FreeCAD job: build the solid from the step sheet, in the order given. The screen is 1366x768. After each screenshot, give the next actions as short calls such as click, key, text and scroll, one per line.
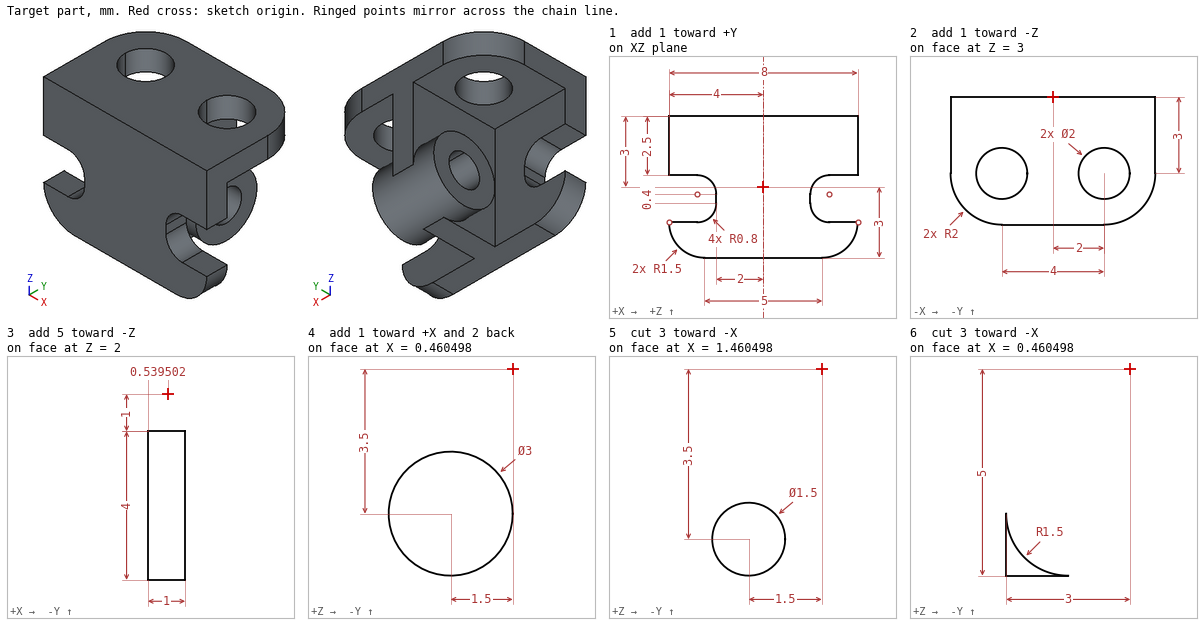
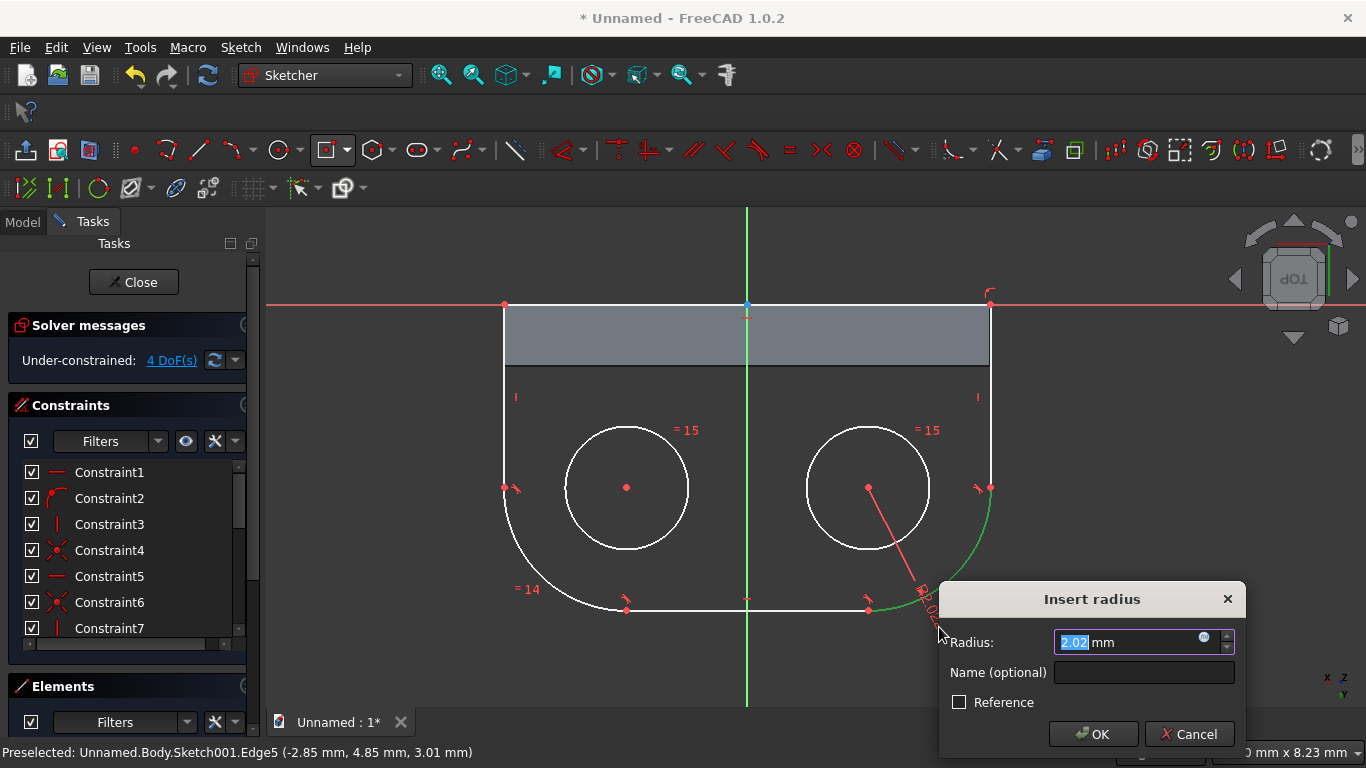
text(2)
key(Return)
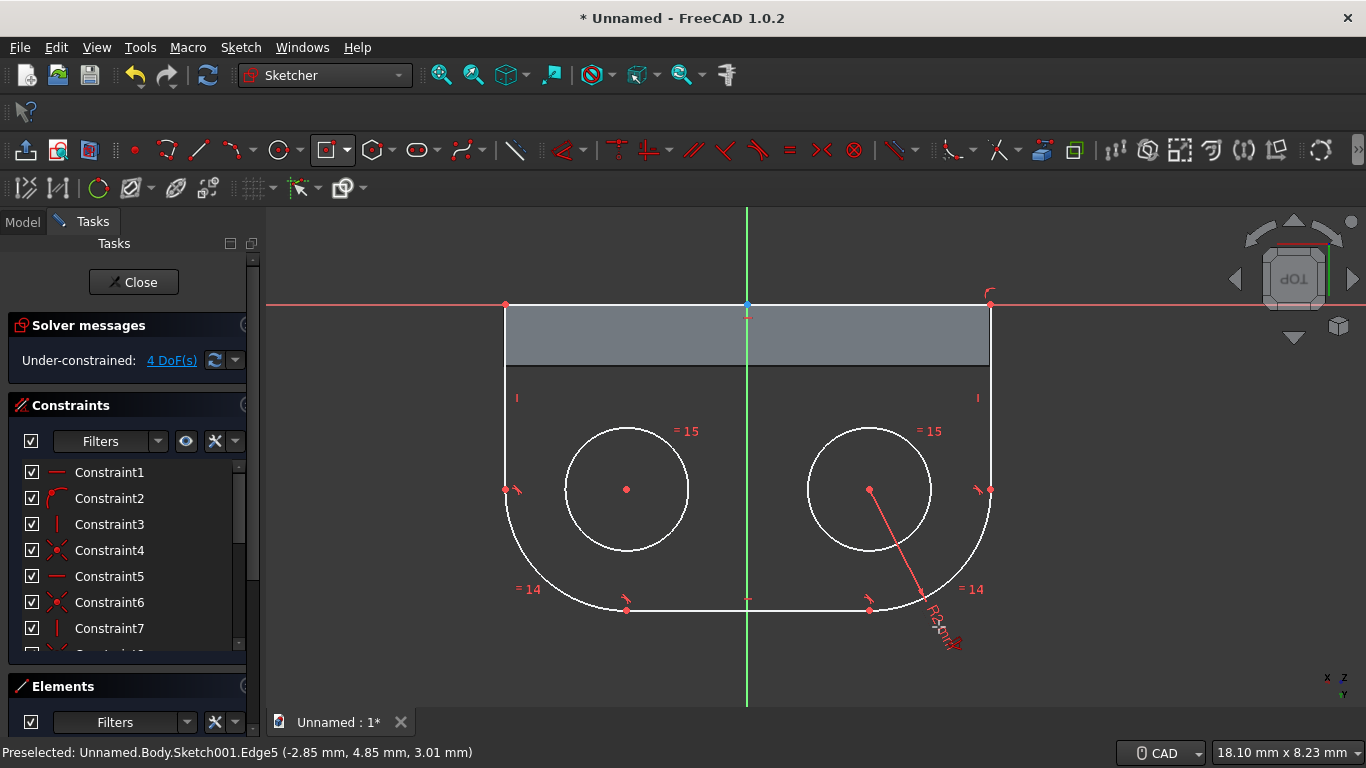
click(913, 446)
click(936, 423)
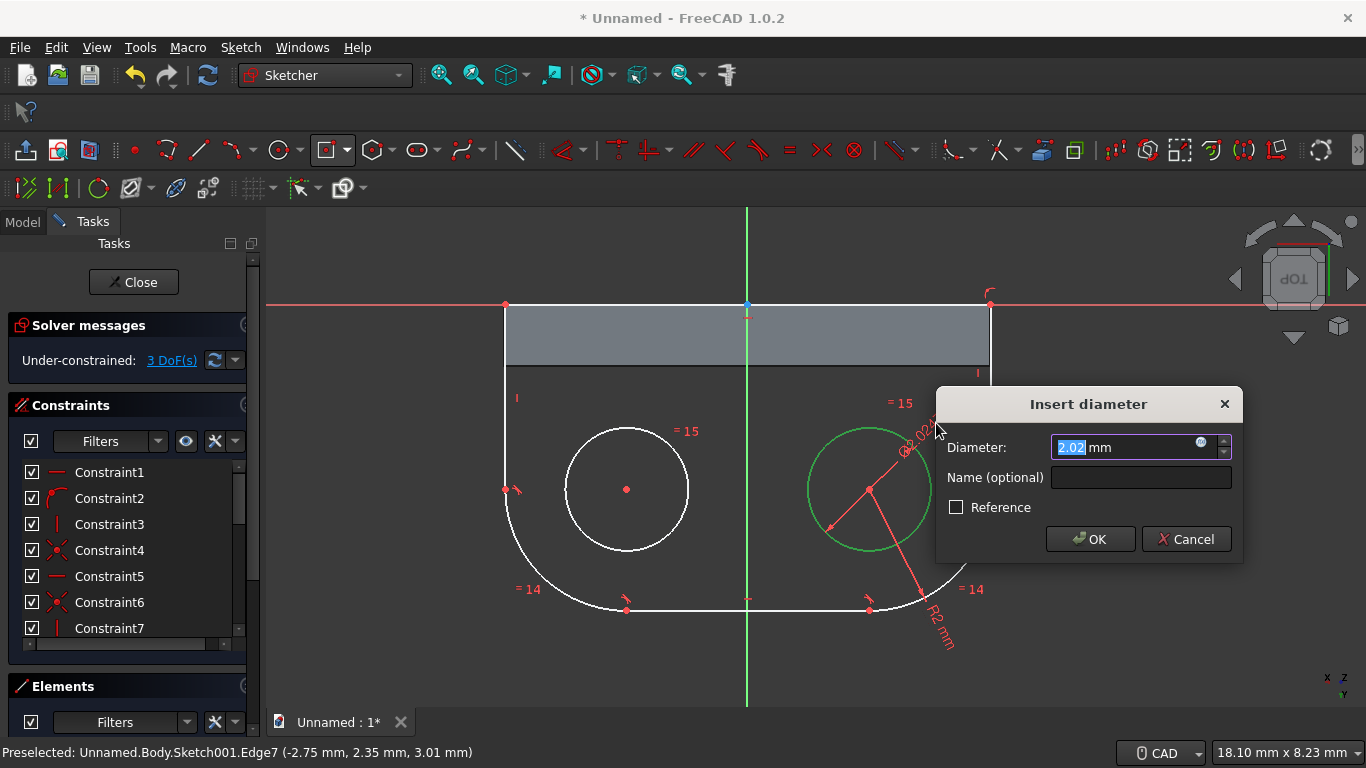
text(2)
key(Return)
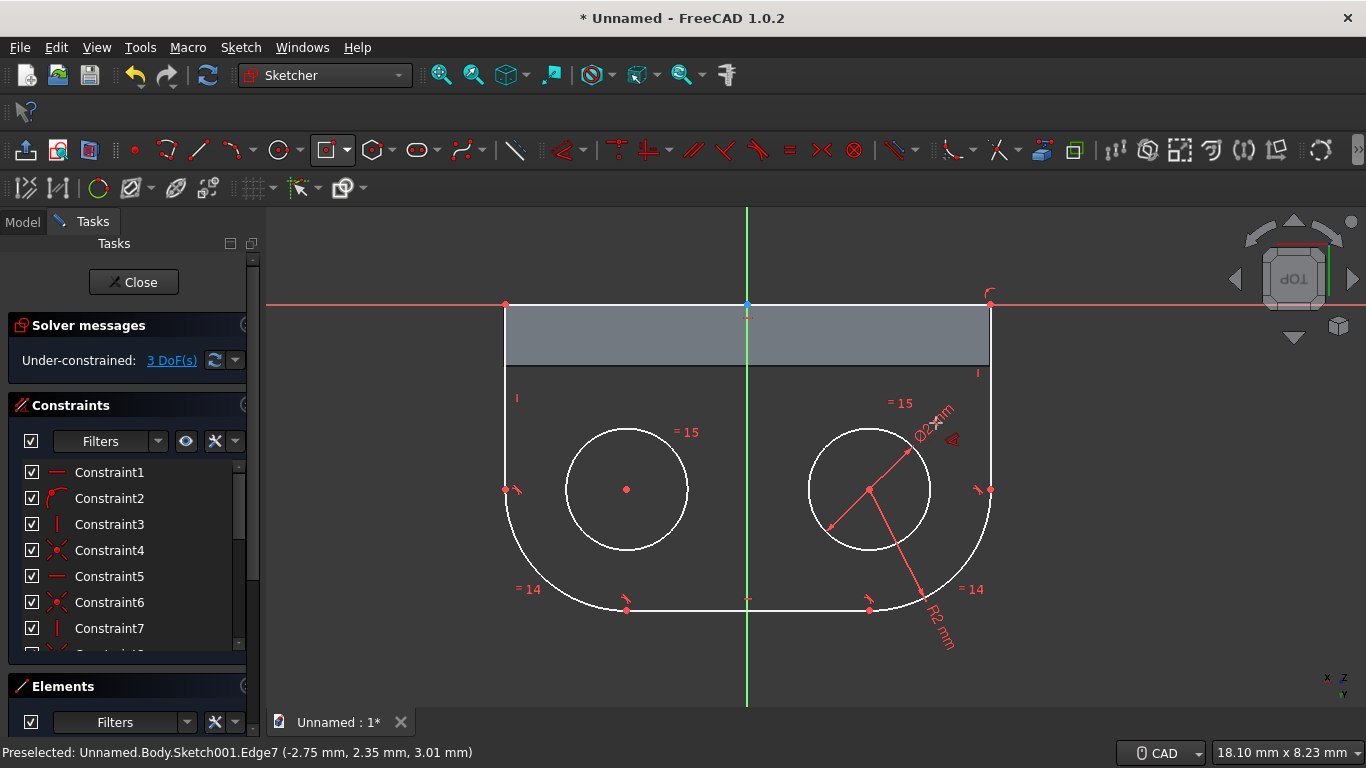
click(700, 611)
click(692, 645)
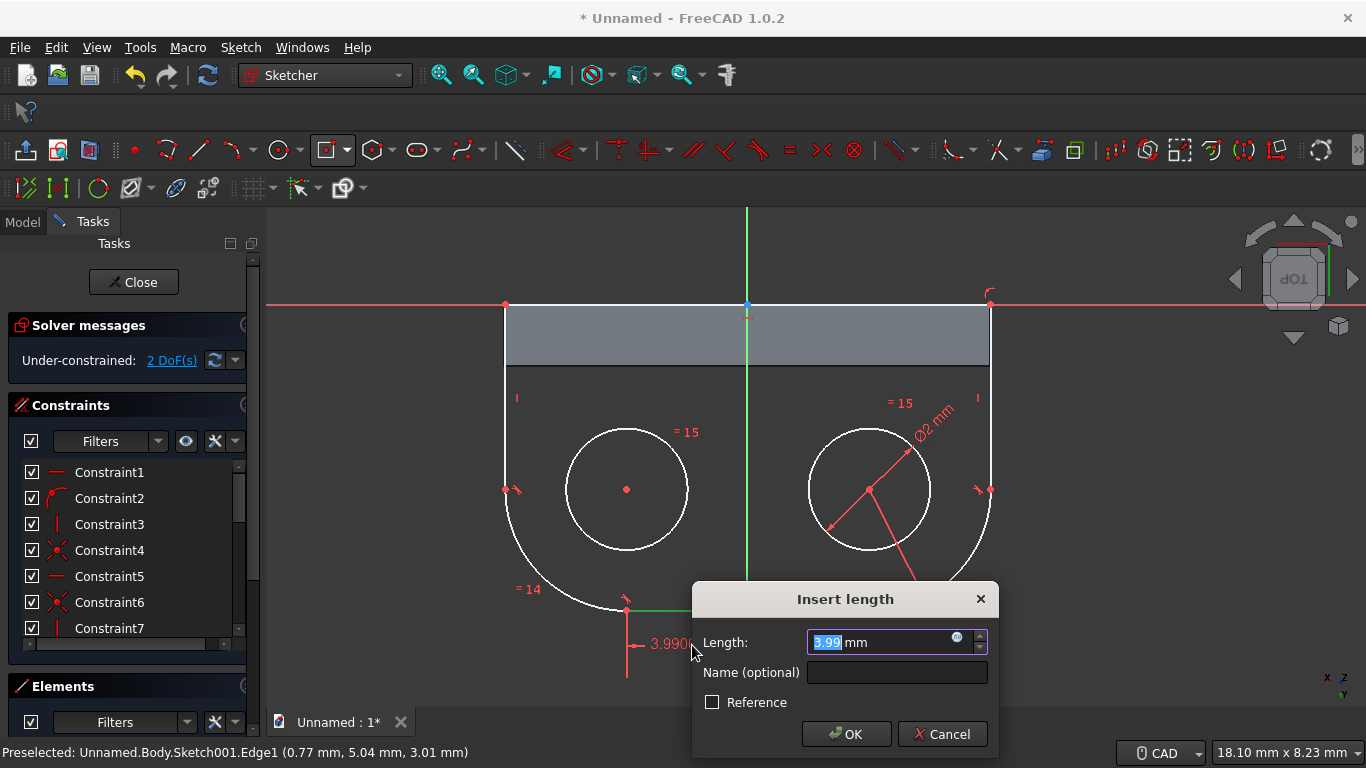
text(4)
key(Return)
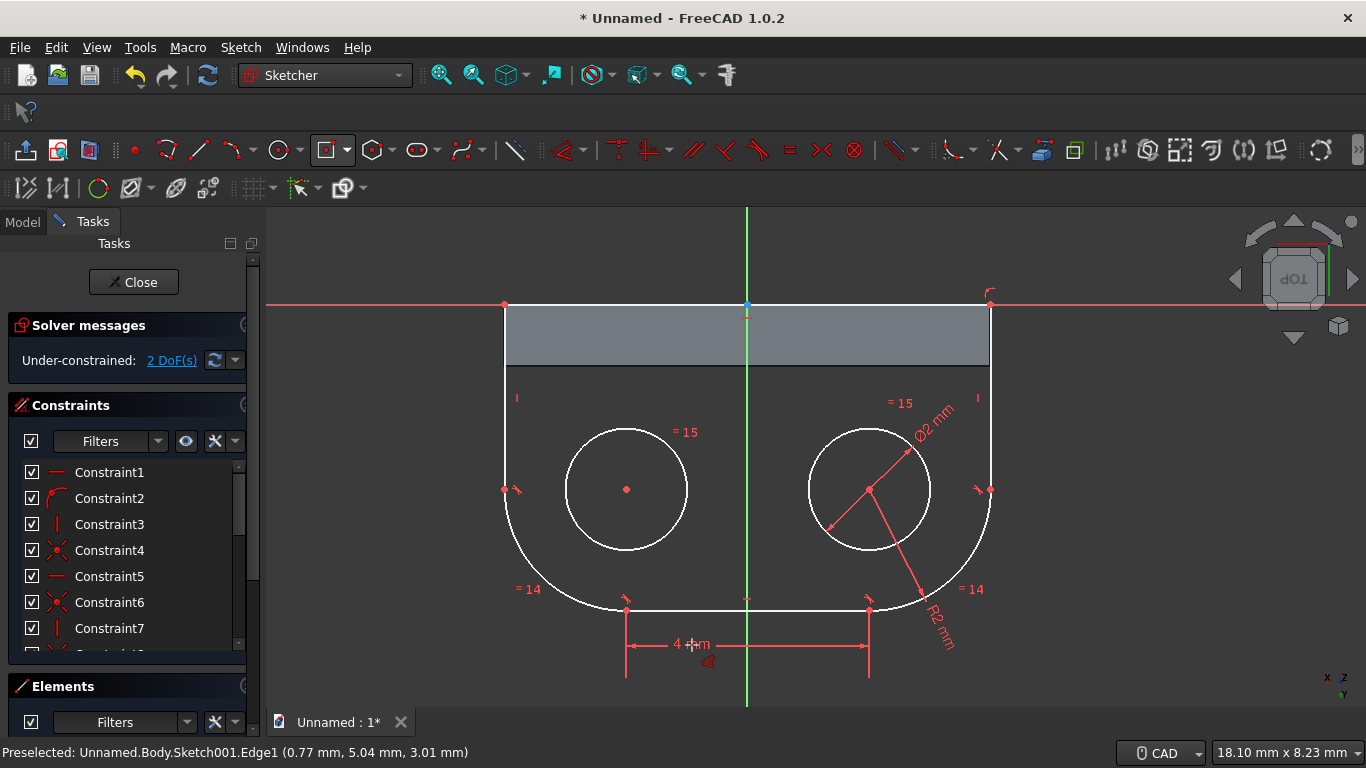
click(991, 434)
click(1025, 397)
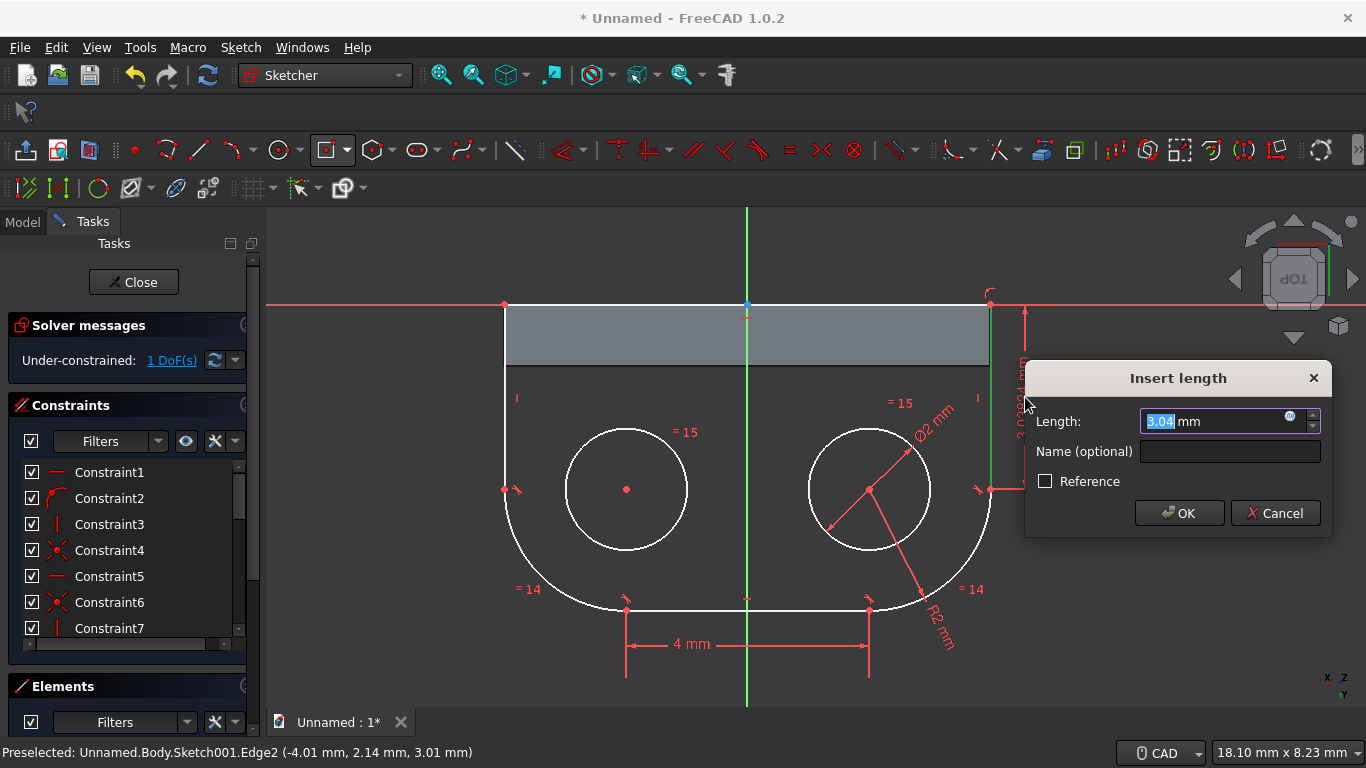
text(3)
key(Return)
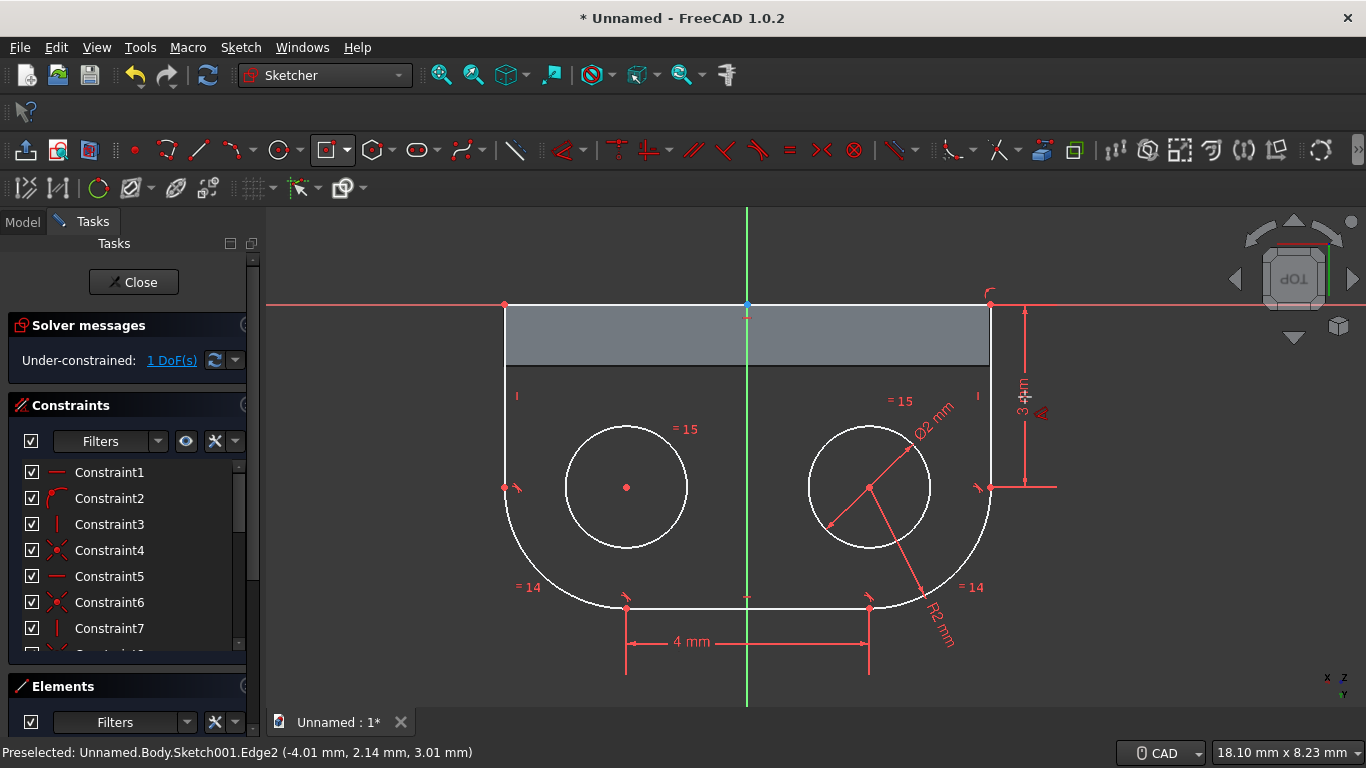
click(869, 487)
click(808, 271)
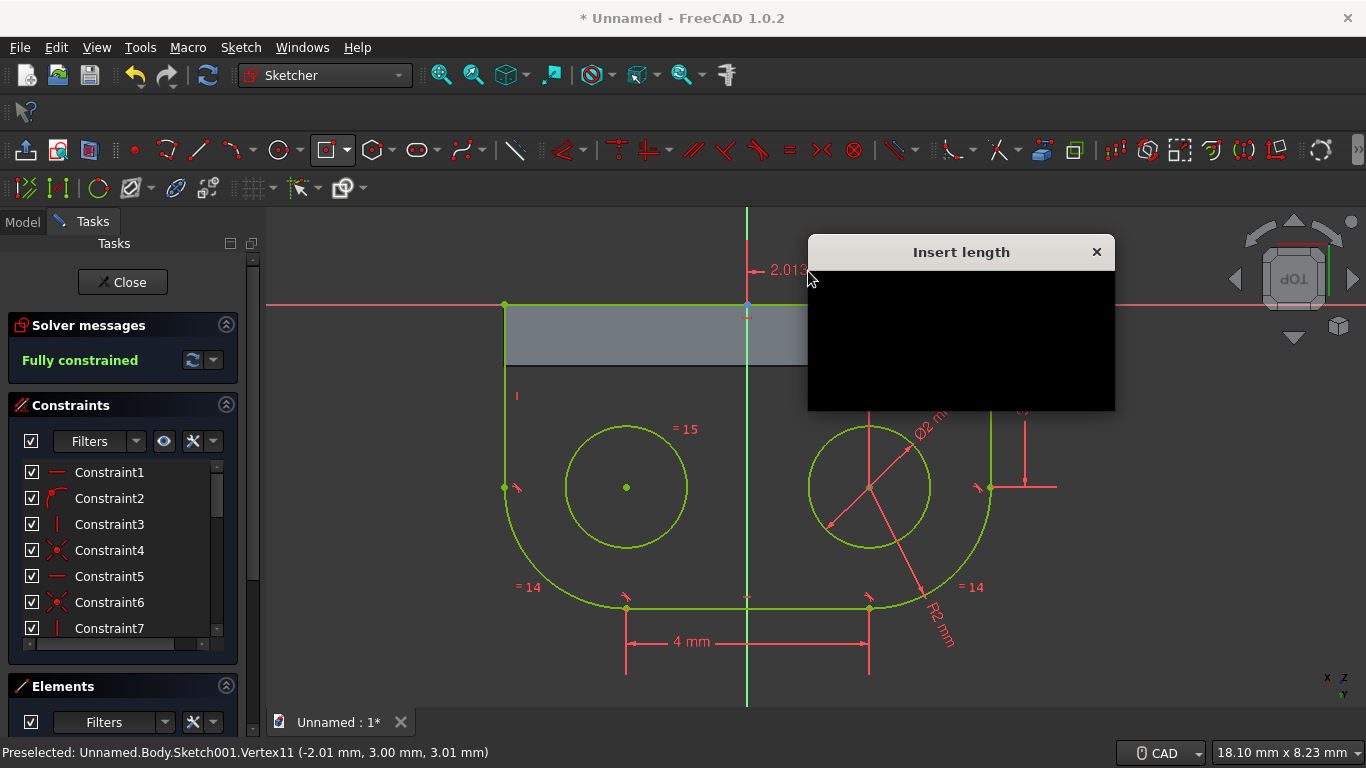
text(2)
key(Return)
key(Escape)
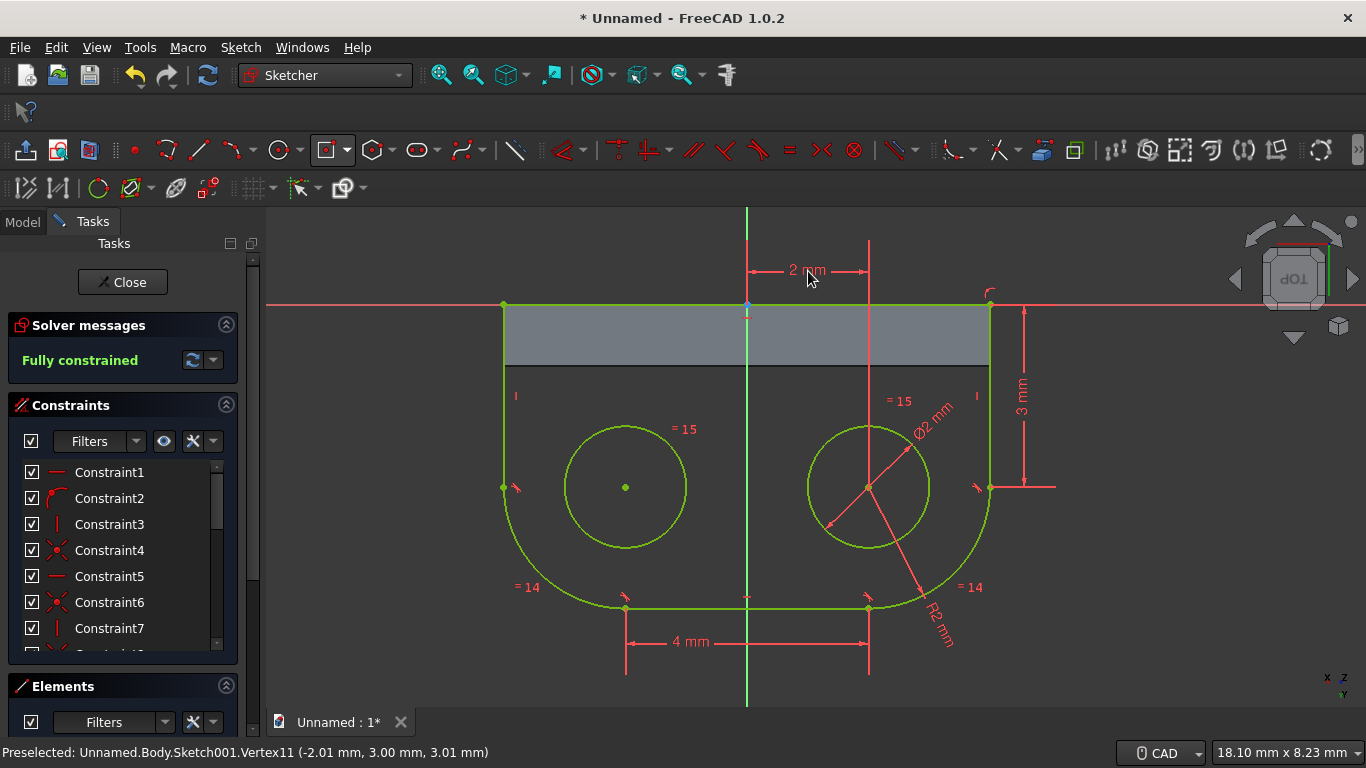
click(123, 282)